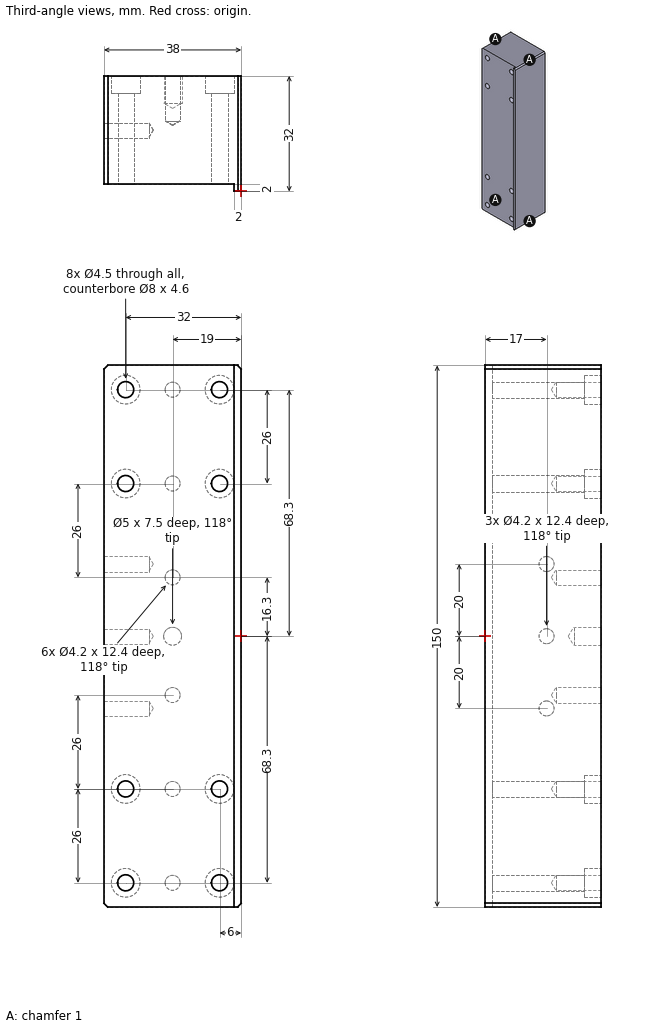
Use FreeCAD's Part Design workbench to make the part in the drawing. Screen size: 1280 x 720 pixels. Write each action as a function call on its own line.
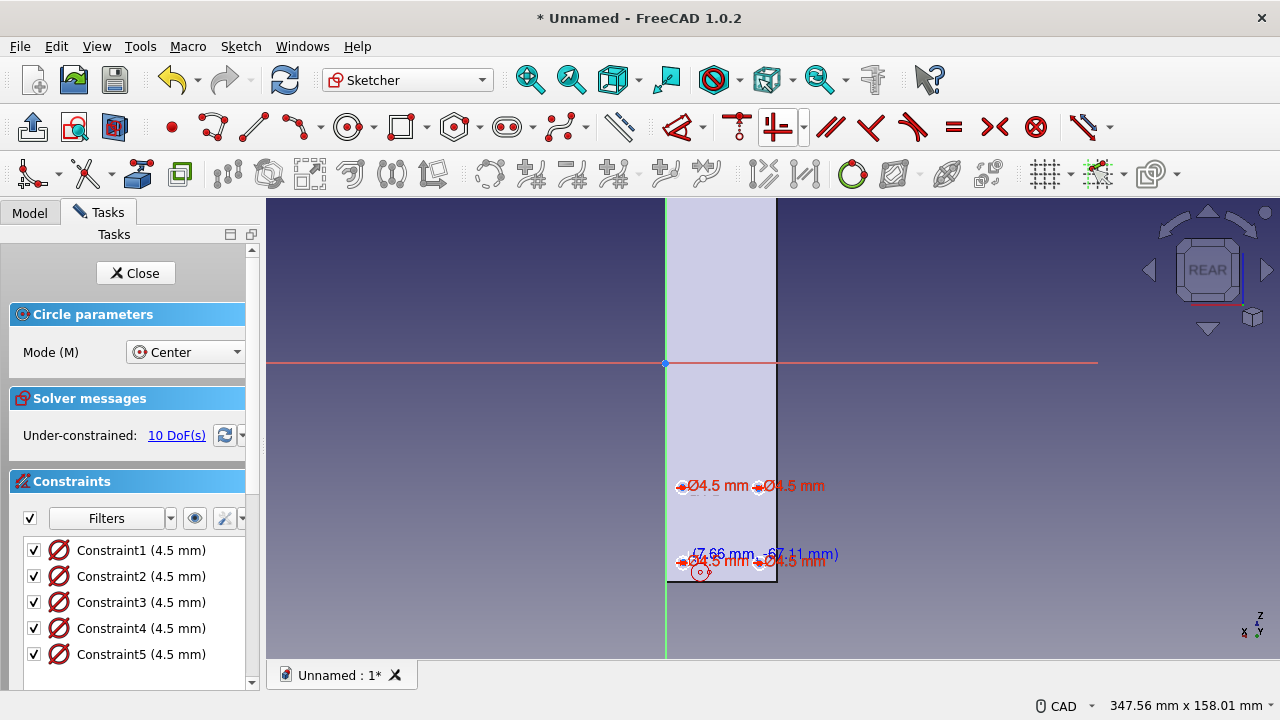
scroll(682, 561, down, 2)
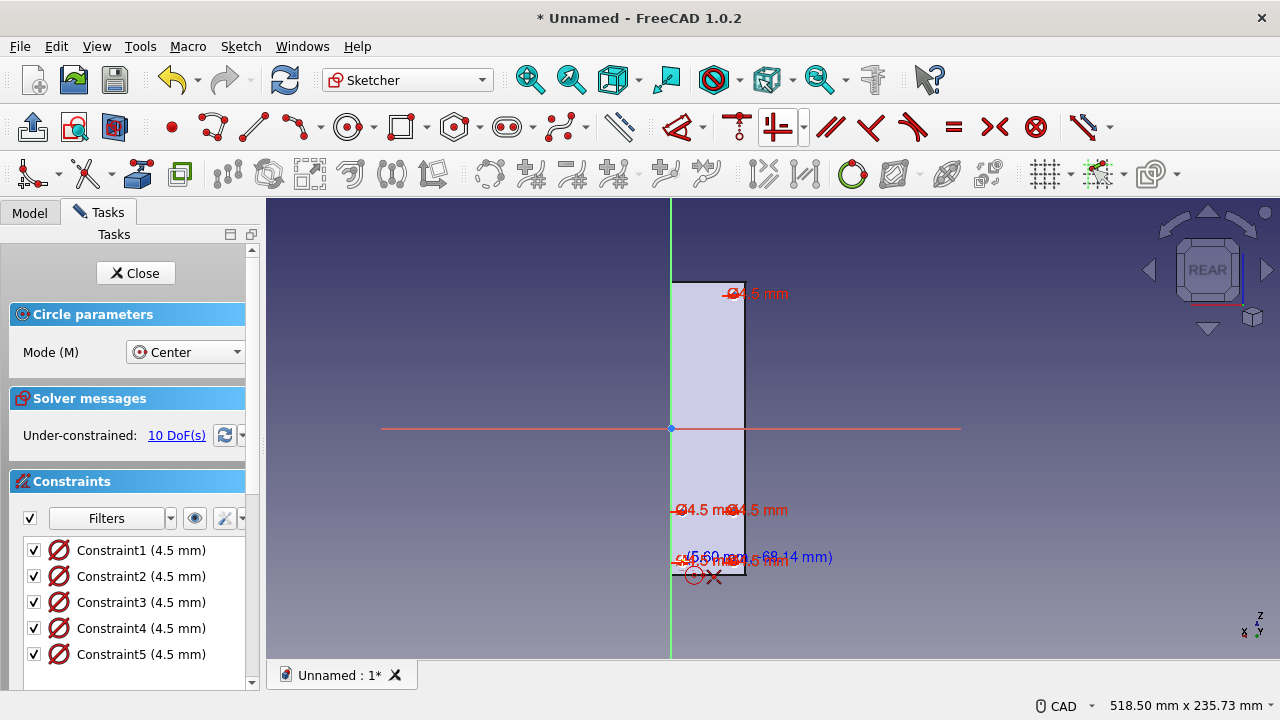
scroll(683, 295, up, 9)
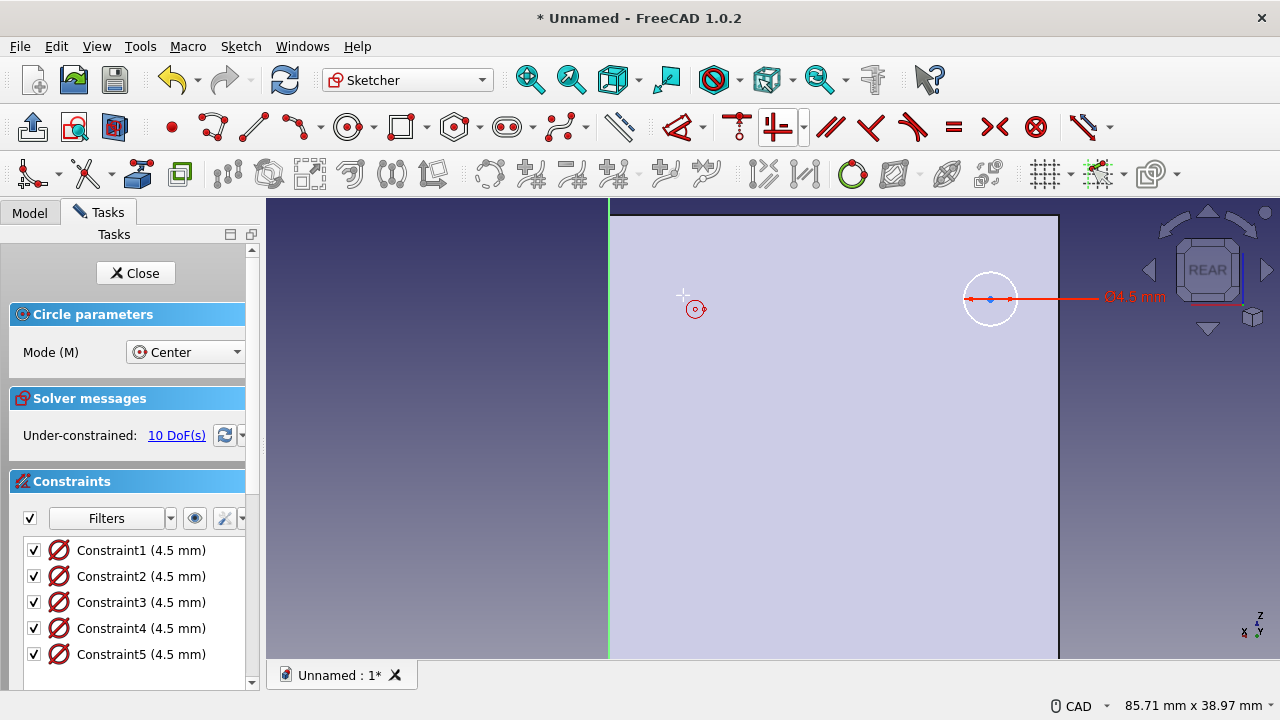
scroll(683, 295, down, 9)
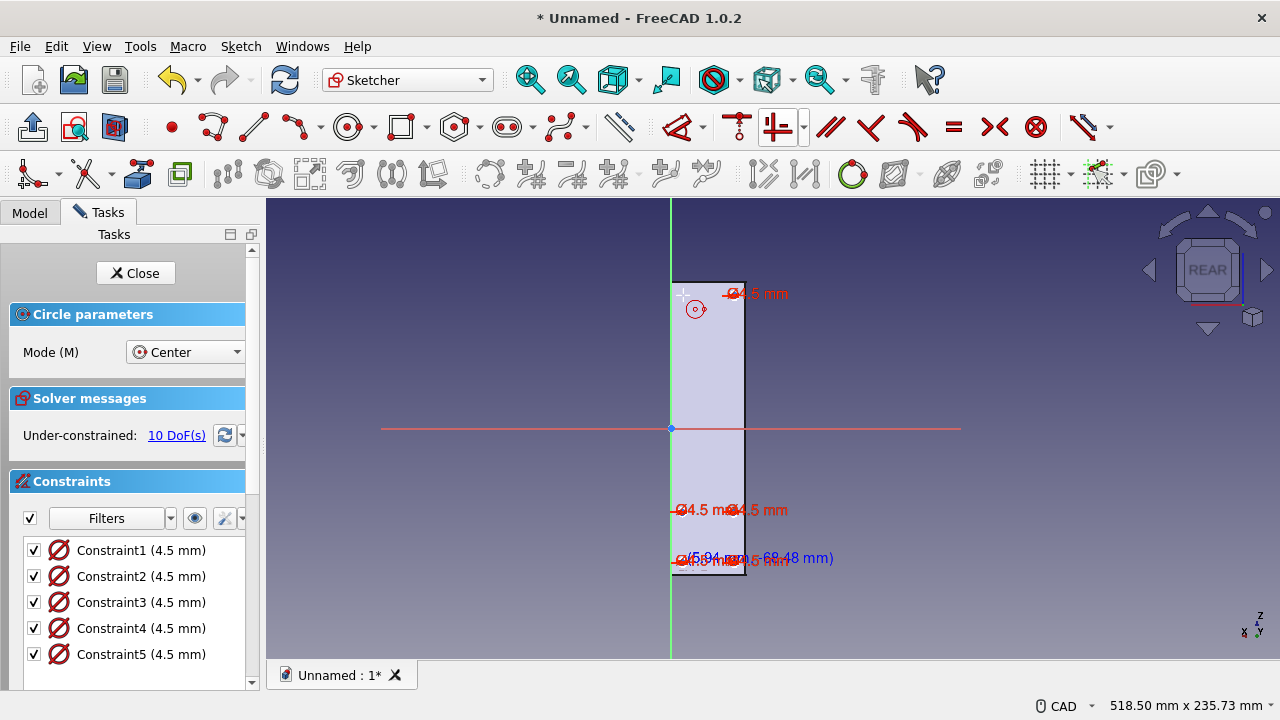
scroll(683, 295, up, 2)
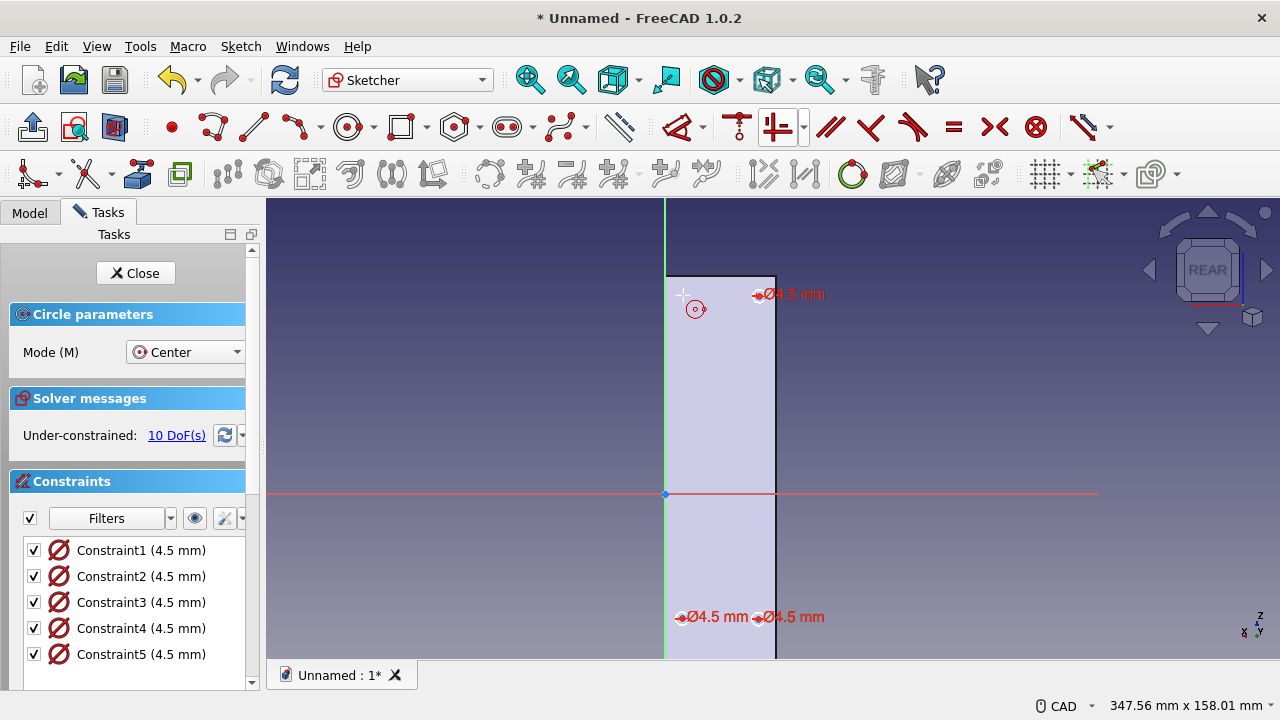
click(683, 295)
move(687, 290)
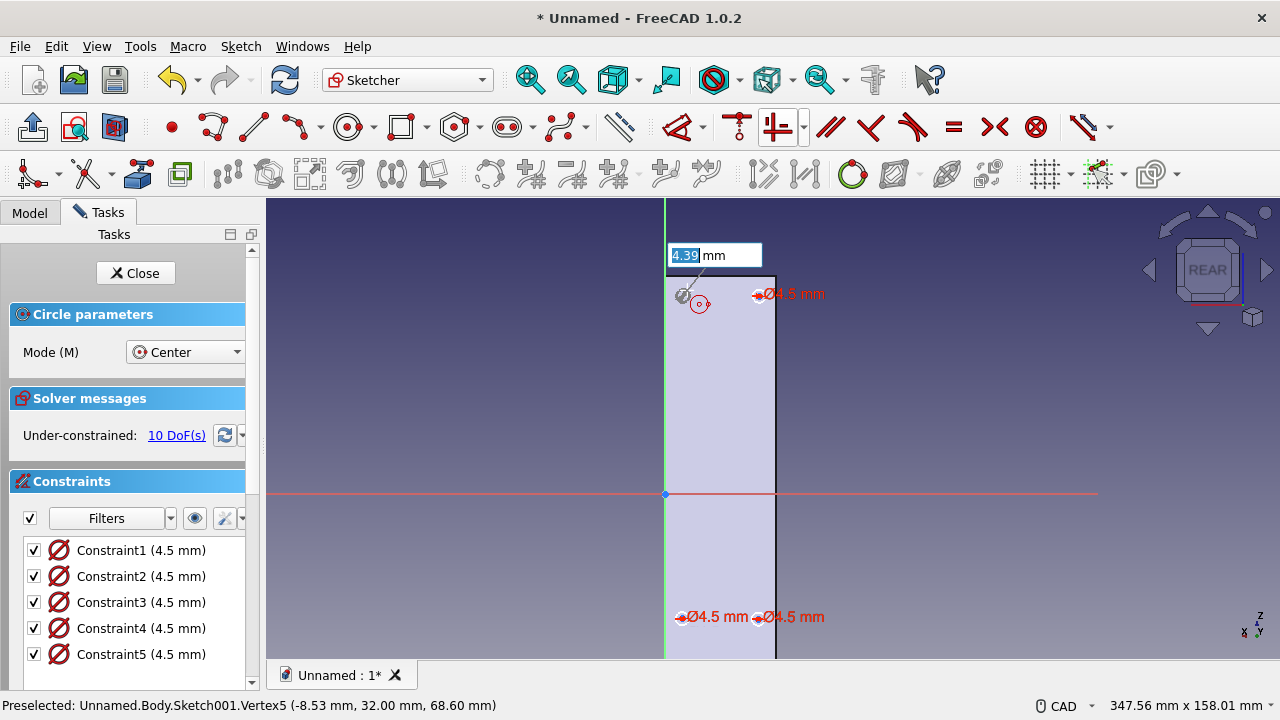
text(4.5)
key(Return)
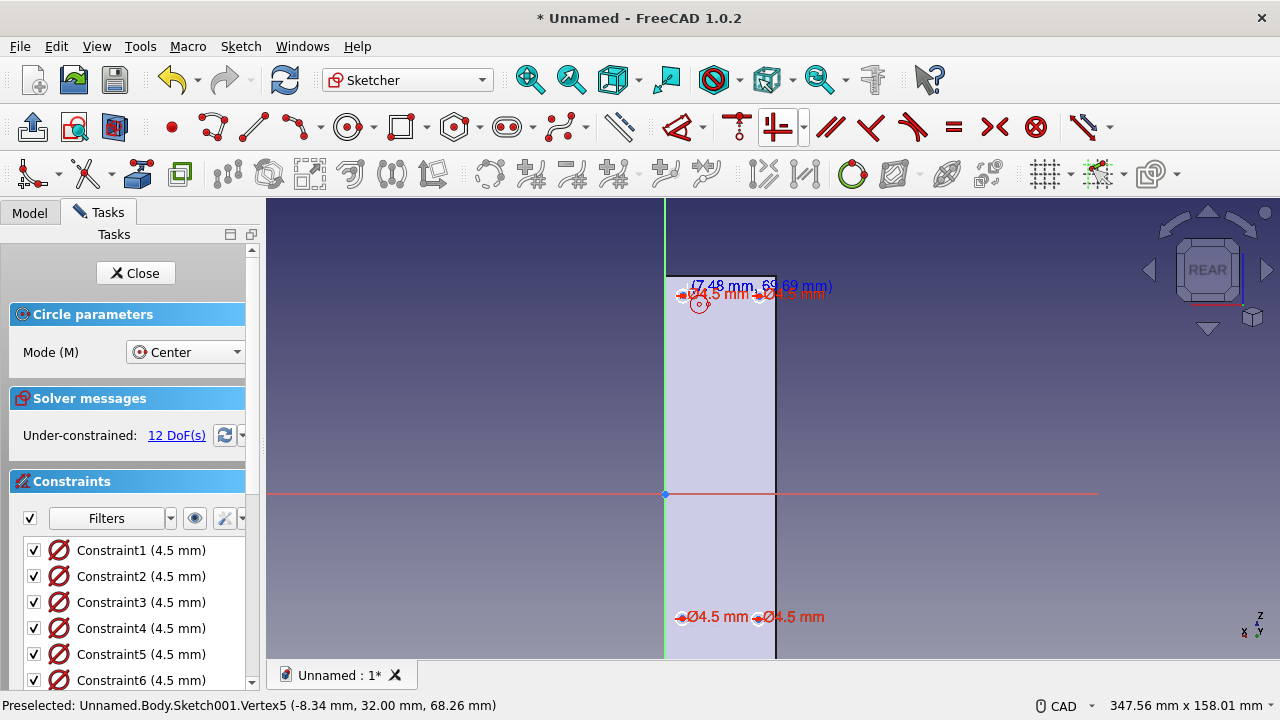
scroll(683, 371, up, 7)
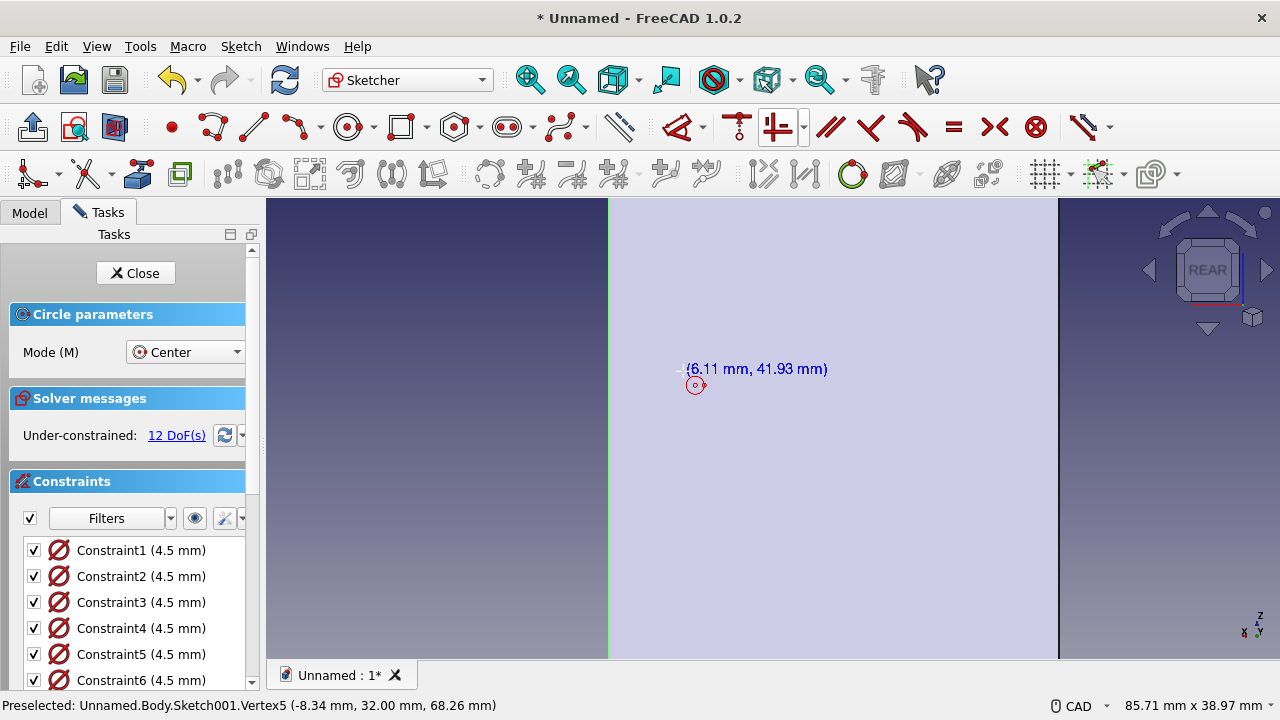
scroll(683, 341, down, 9)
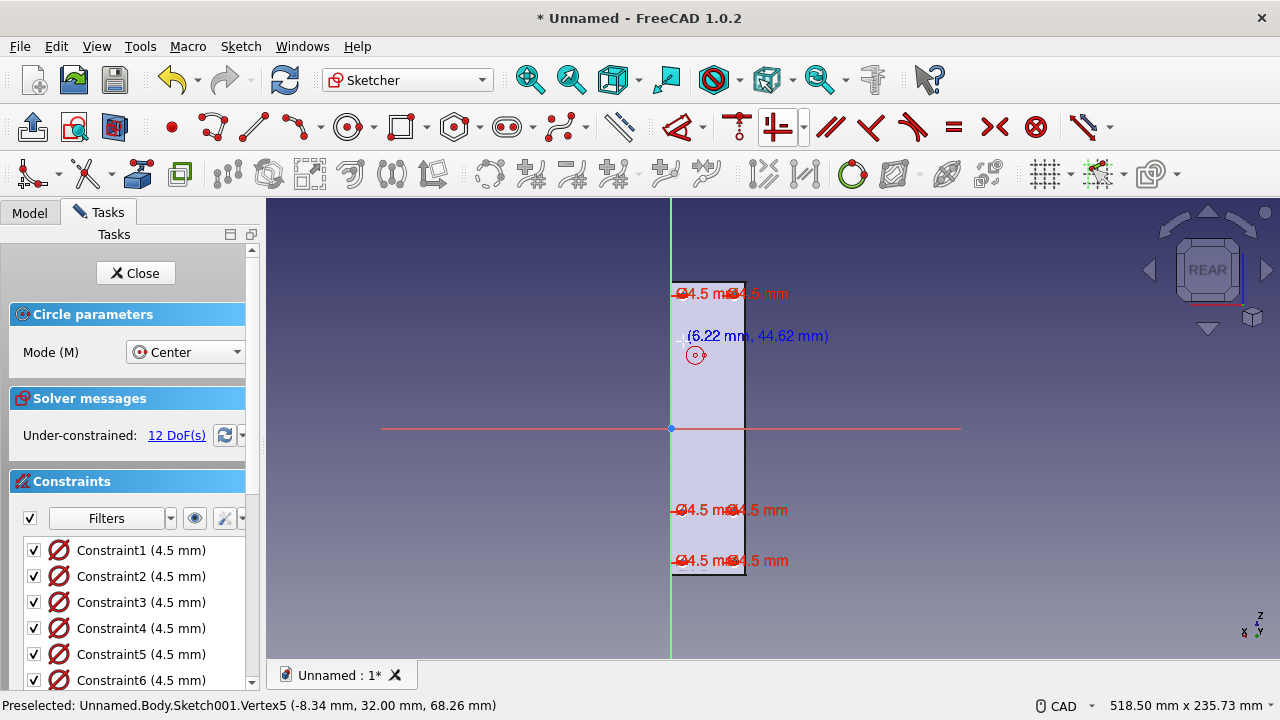
scroll(683, 346, up, 2)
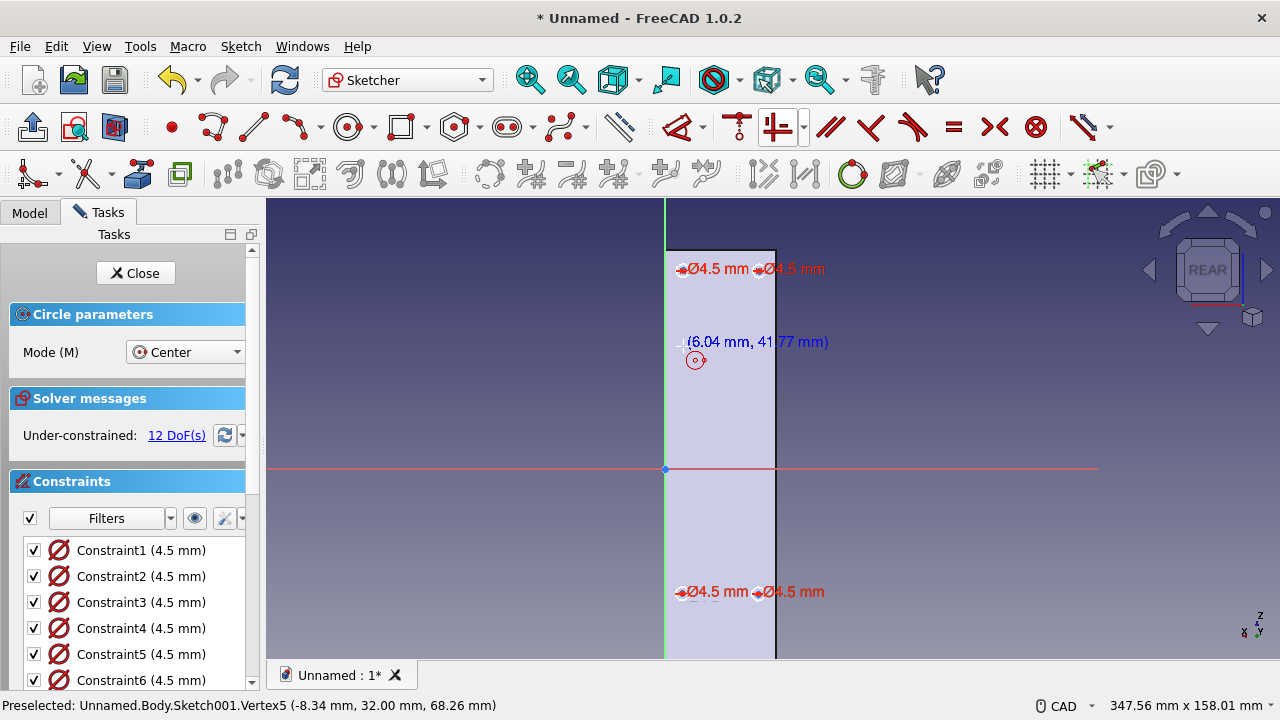
click(683, 346)
move(687, 341)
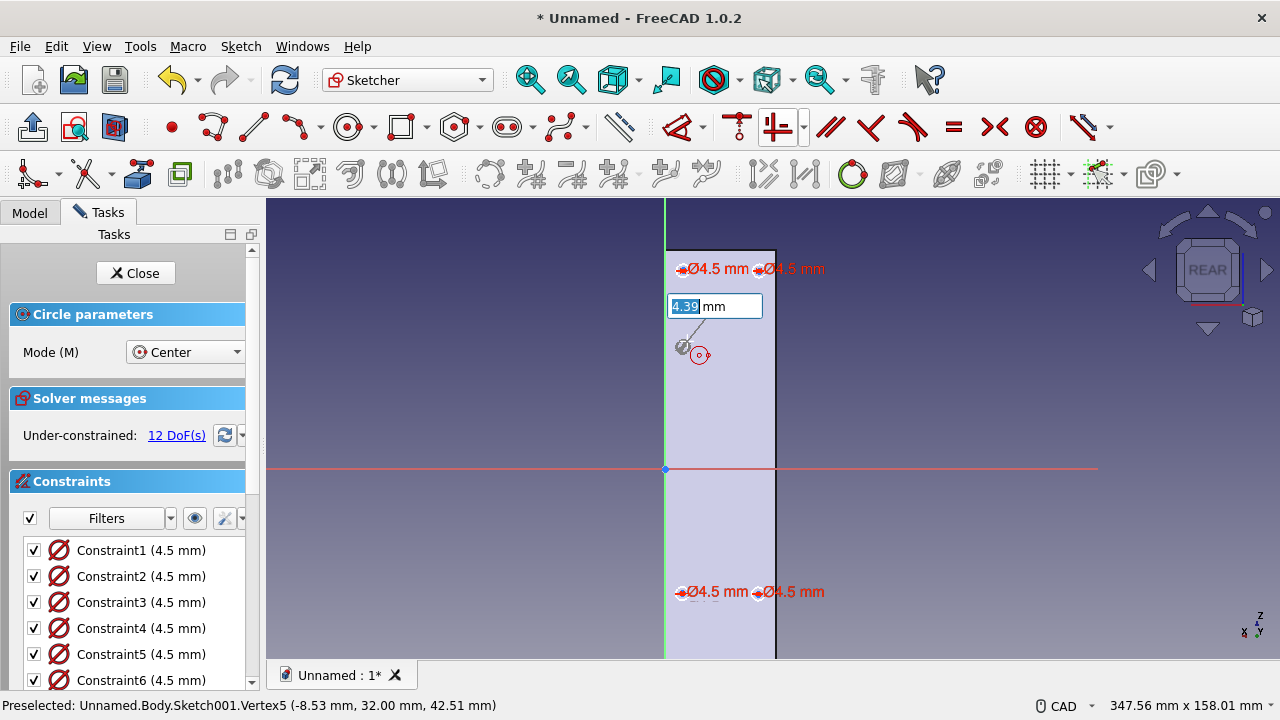
text(4.5)
key(Return)